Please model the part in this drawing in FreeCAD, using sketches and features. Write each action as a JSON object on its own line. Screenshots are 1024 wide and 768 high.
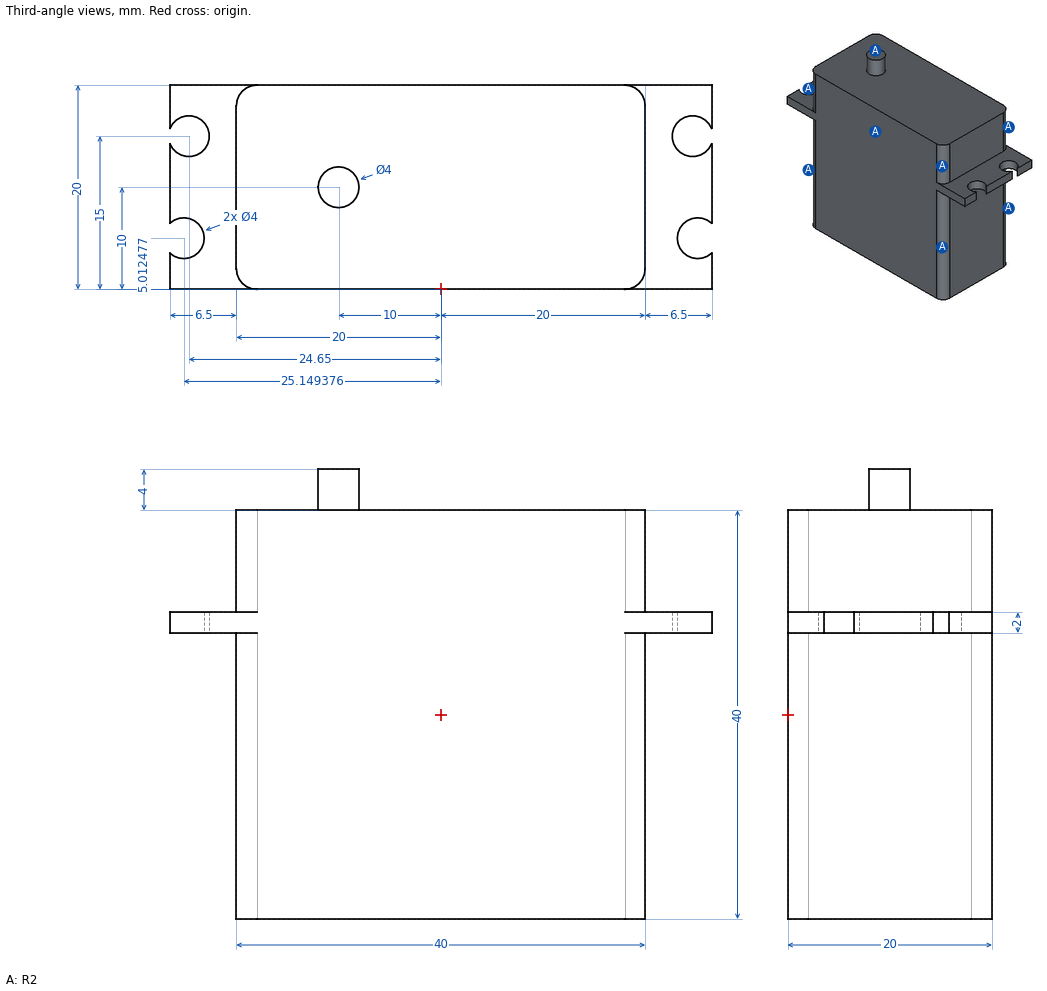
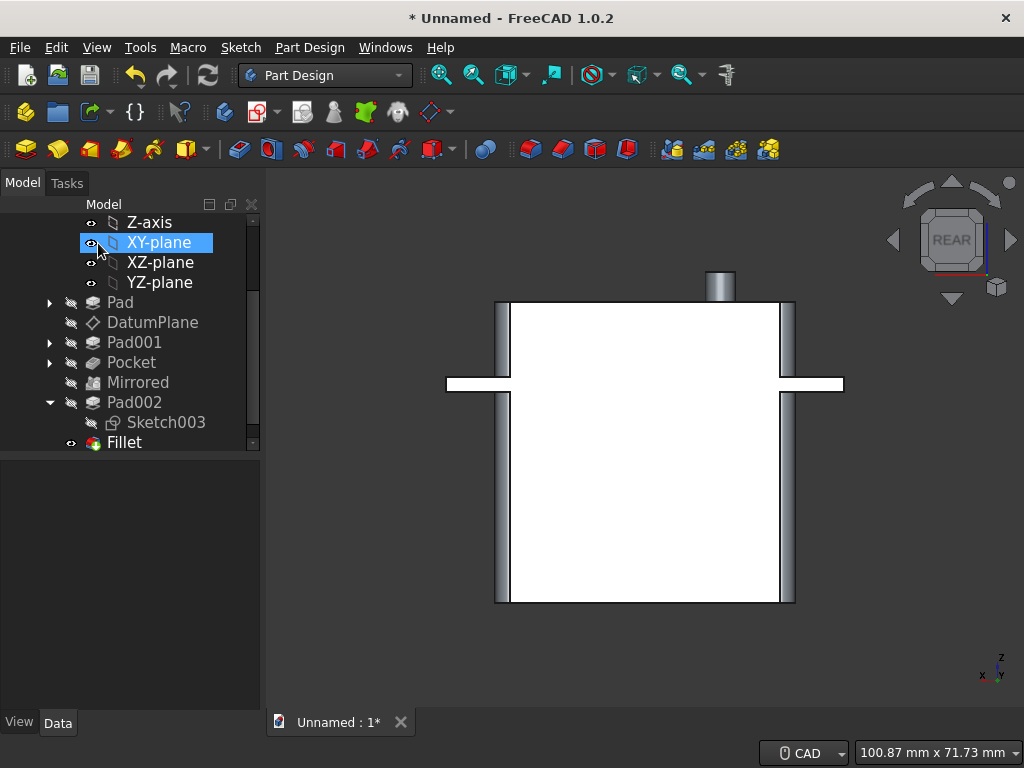
{"action": "key", "text": "0"}